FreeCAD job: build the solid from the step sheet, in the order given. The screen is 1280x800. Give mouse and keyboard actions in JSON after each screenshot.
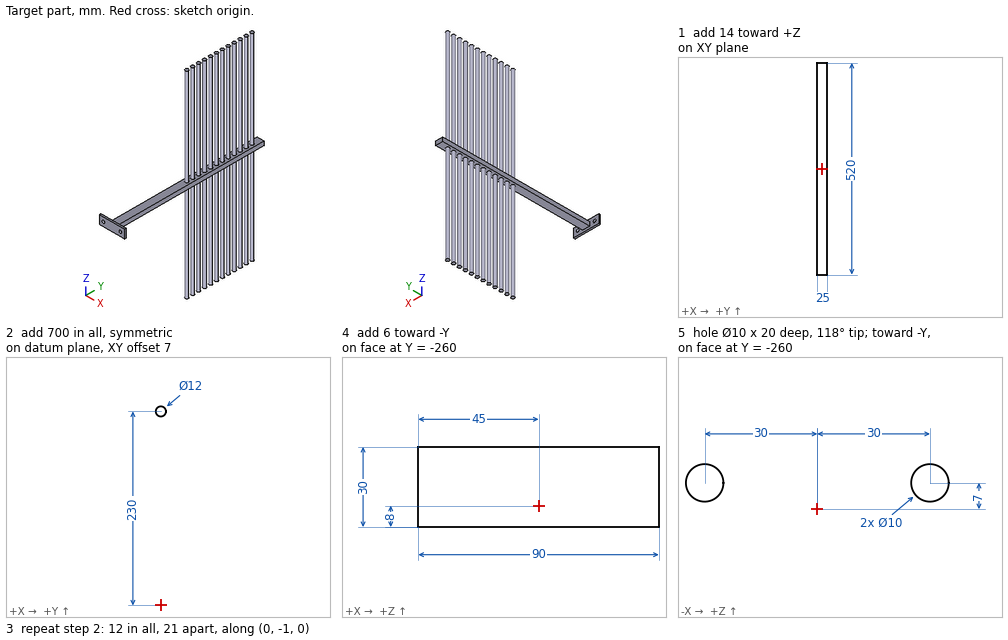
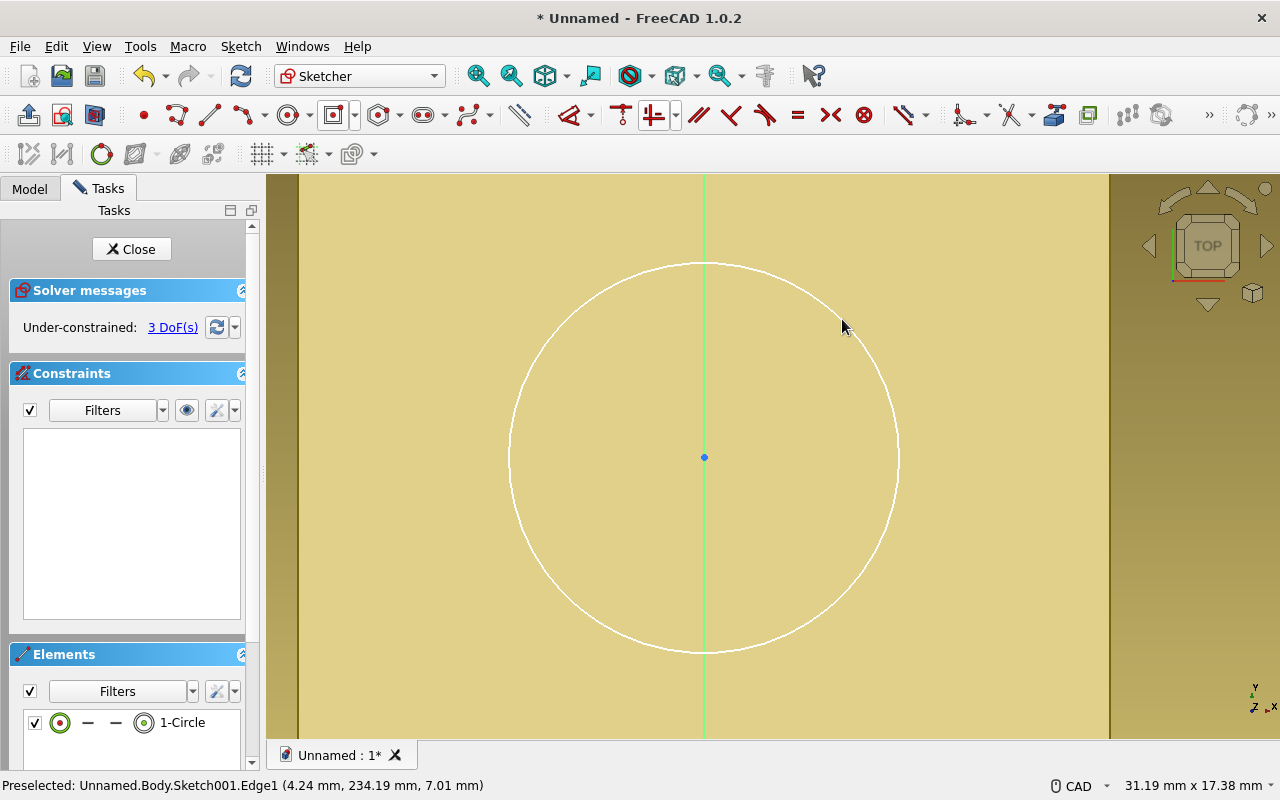
{"action": "left_click", "coordinate": [704, 458]}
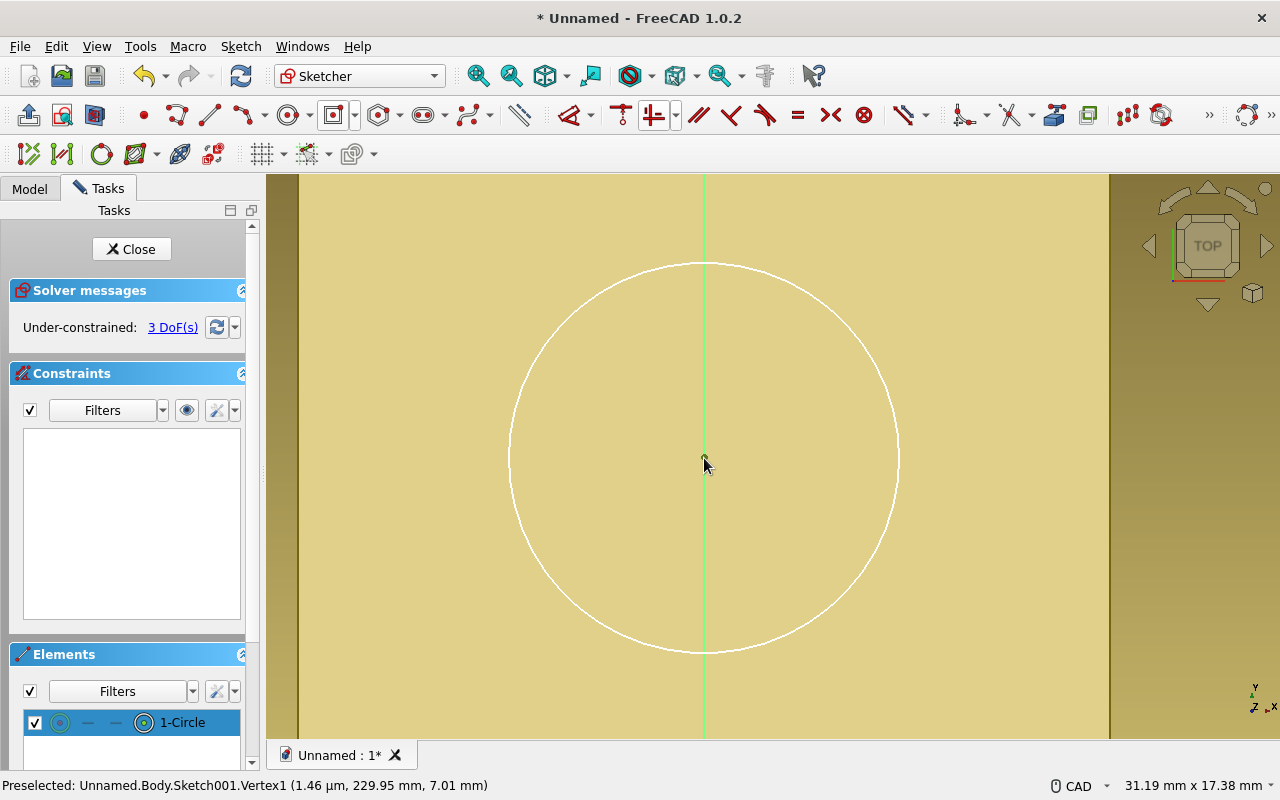
{"action": "left_click", "coordinate": [704, 602]}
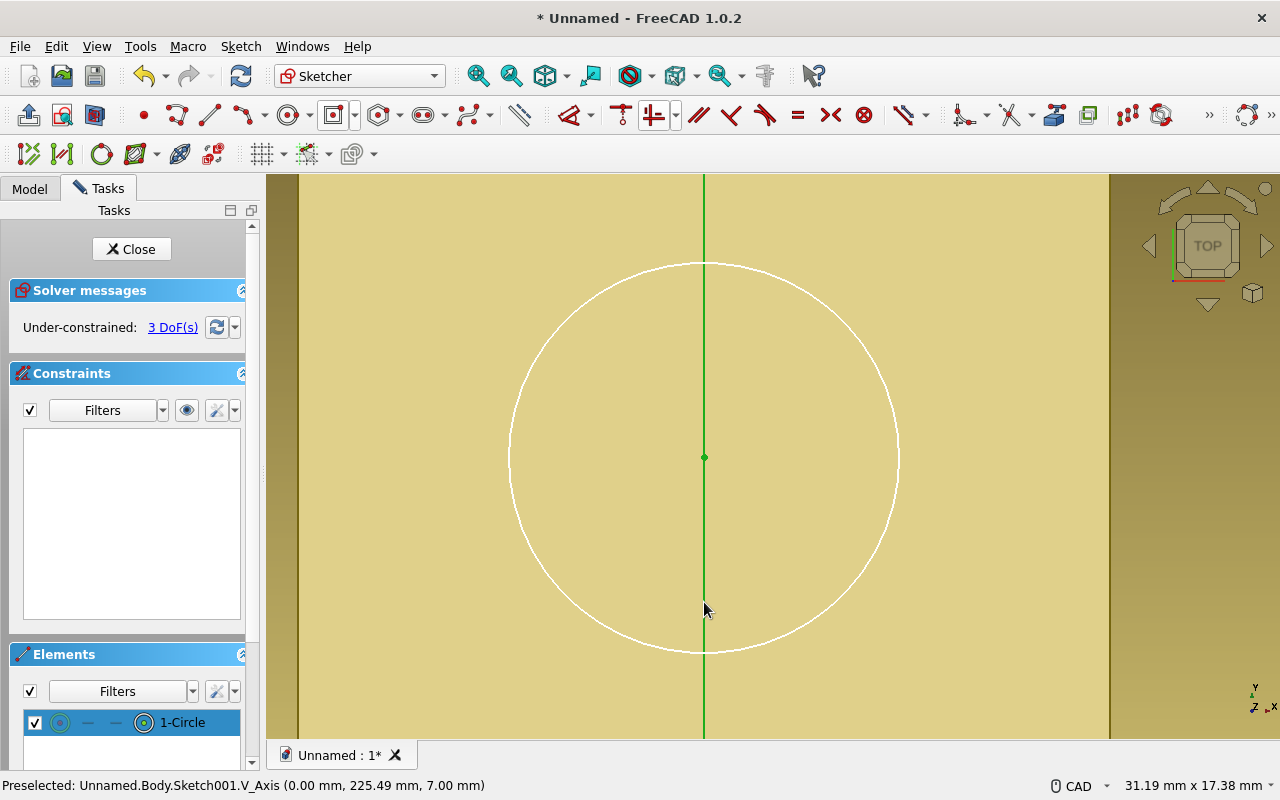
{"action": "left_click", "coordinate": [621, 116]}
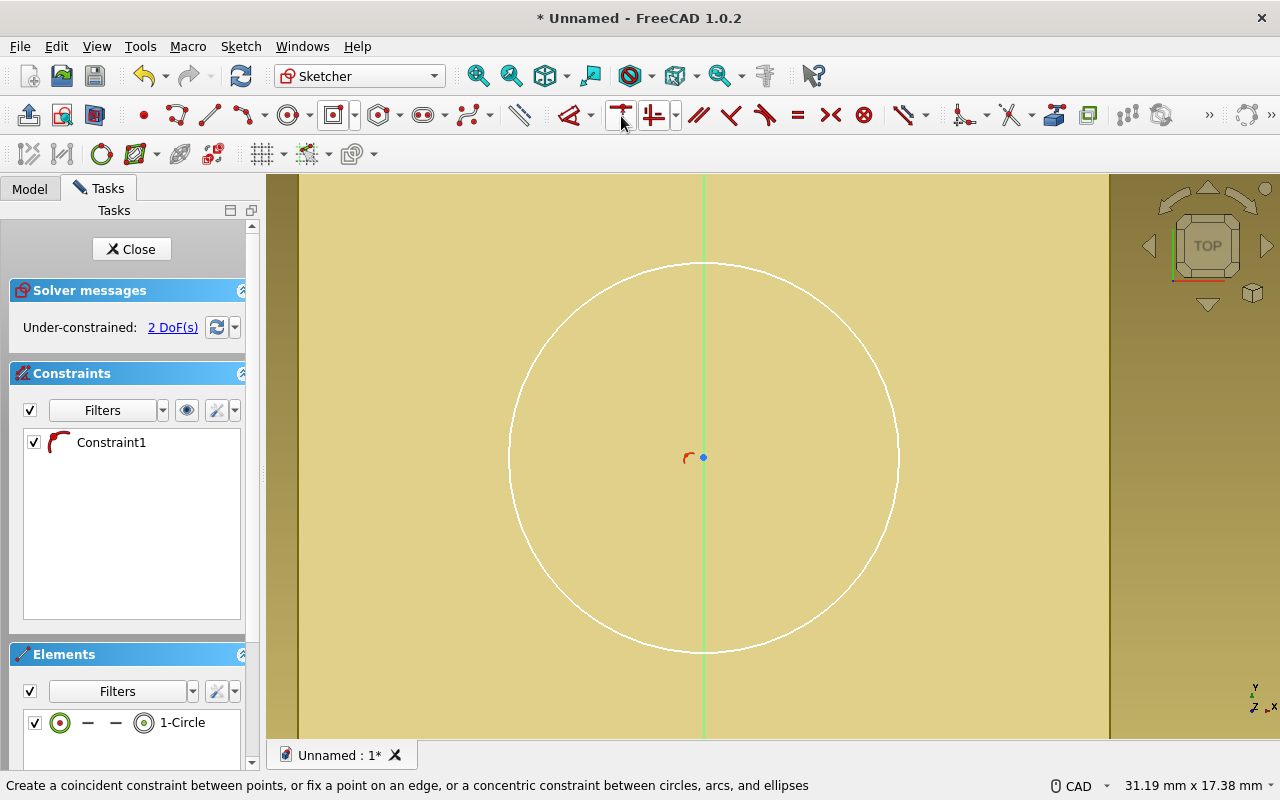
{"action": "left_click", "coordinate": [568, 116]}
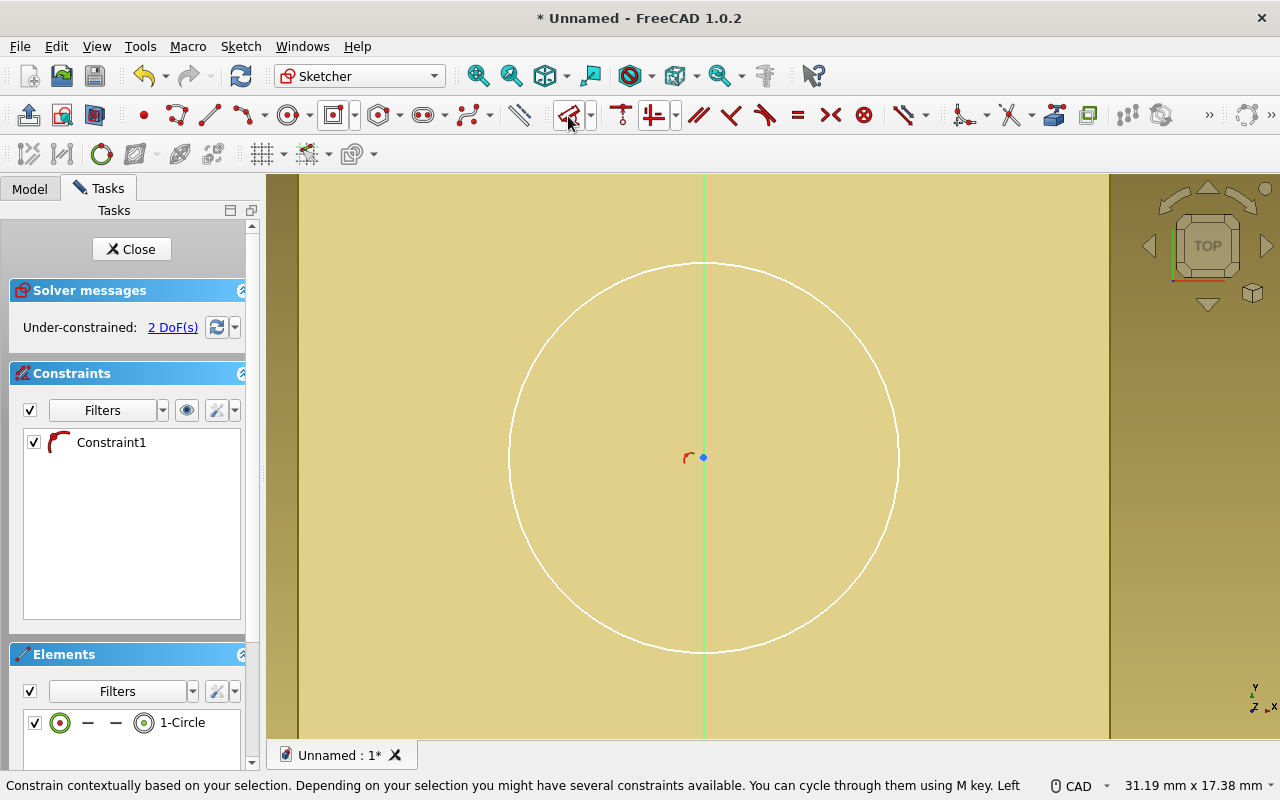
{"action": "left_click", "coordinate": [842, 320]}
{"action": "left_click", "coordinate": [865, 297]}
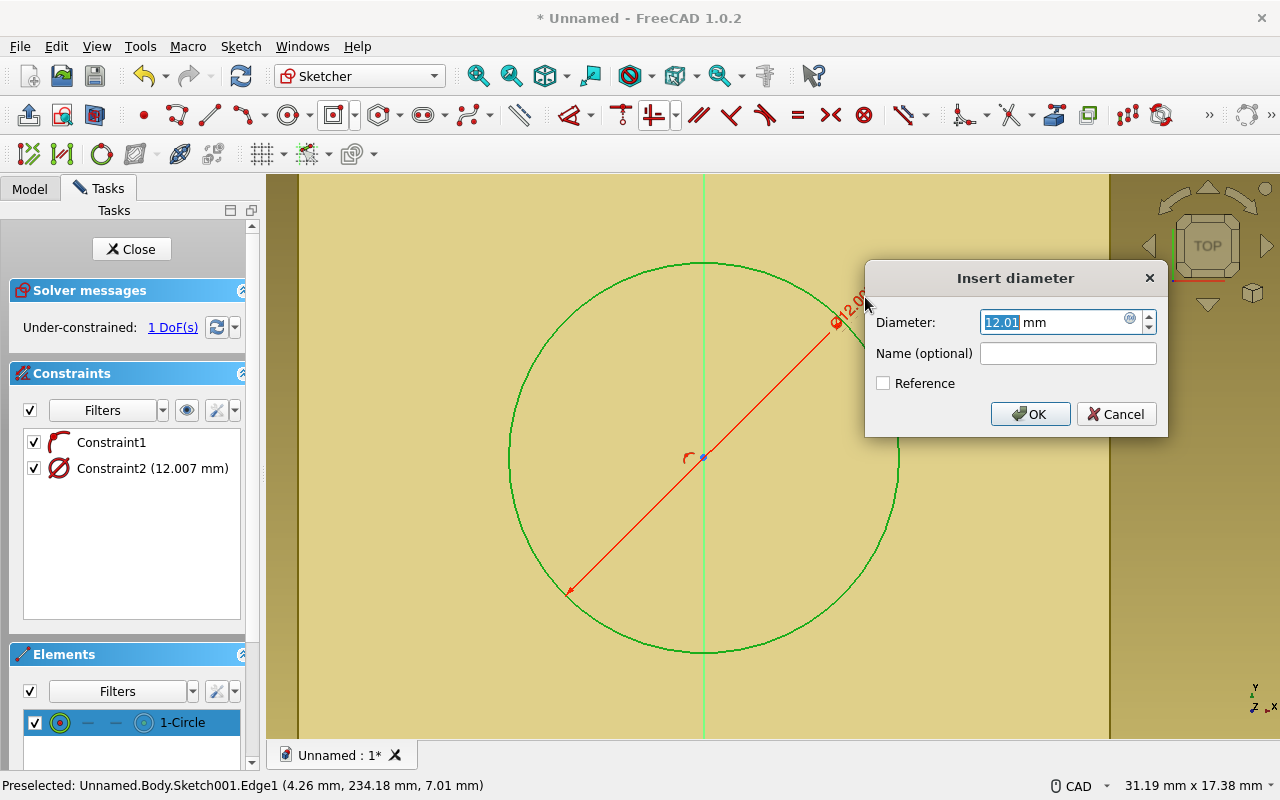
{"action": "type", "text": "12"}
{"action": "key", "text": "Return"}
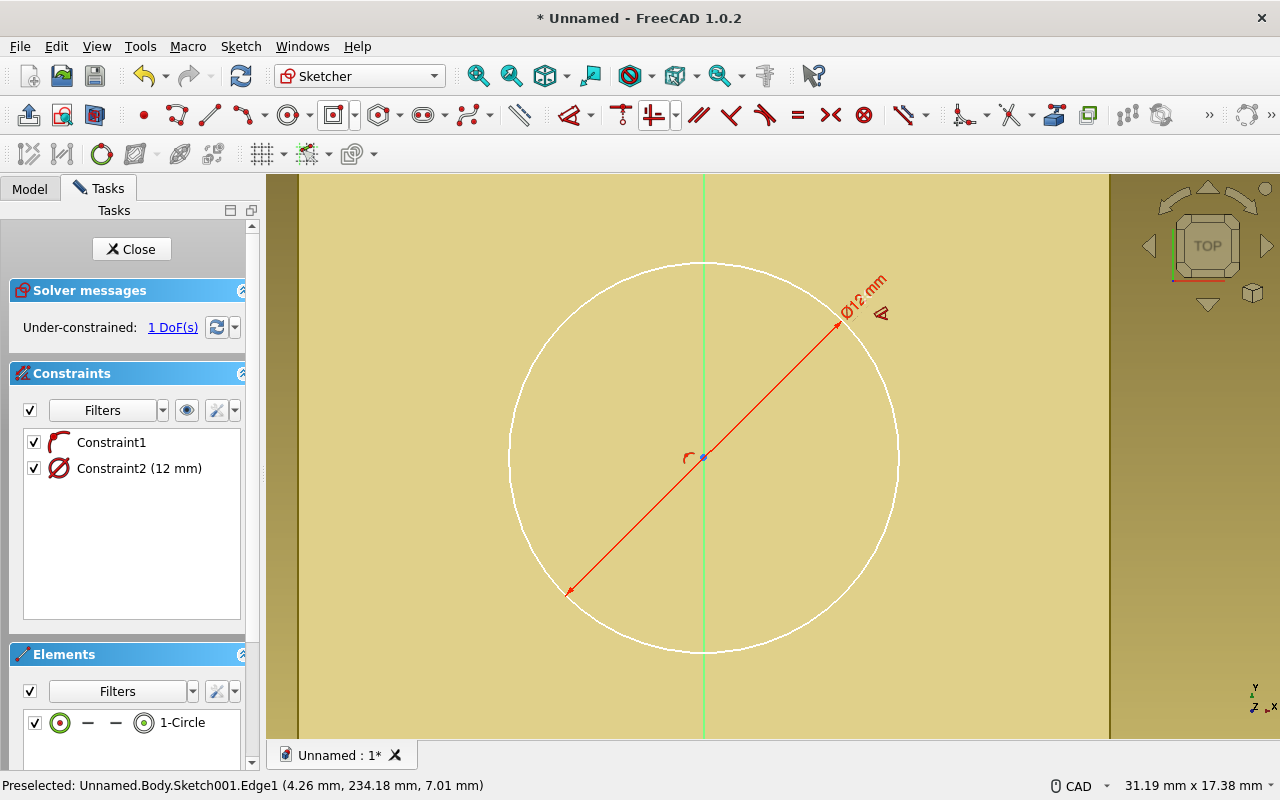
{"action": "left_click", "coordinate": [704, 458]}
{"action": "left_click", "coordinate": [738, 585]}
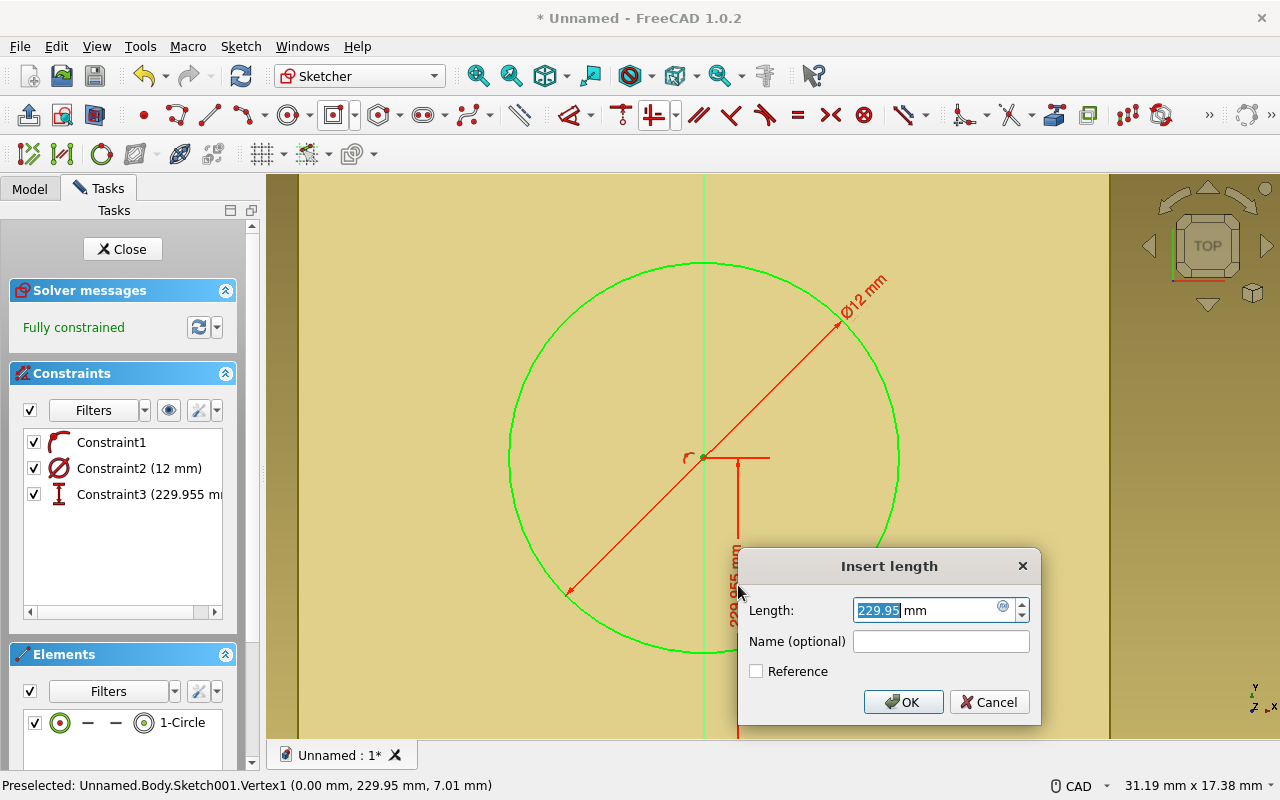
{"action": "type", "text": "230"}
{"action": "key", "text": "Return"}
{"action": "key", "text": "Escape"}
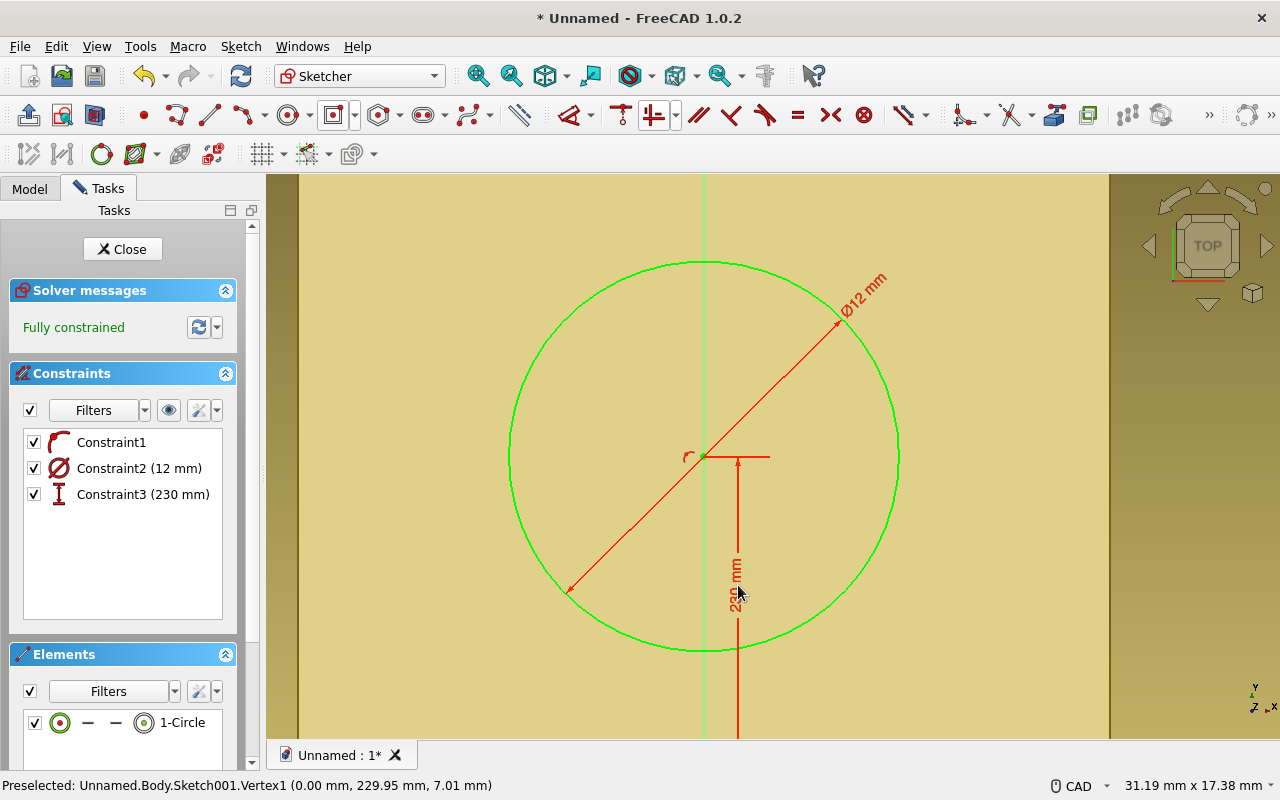
{"action": "left_click", "coordinate": [123, 249]}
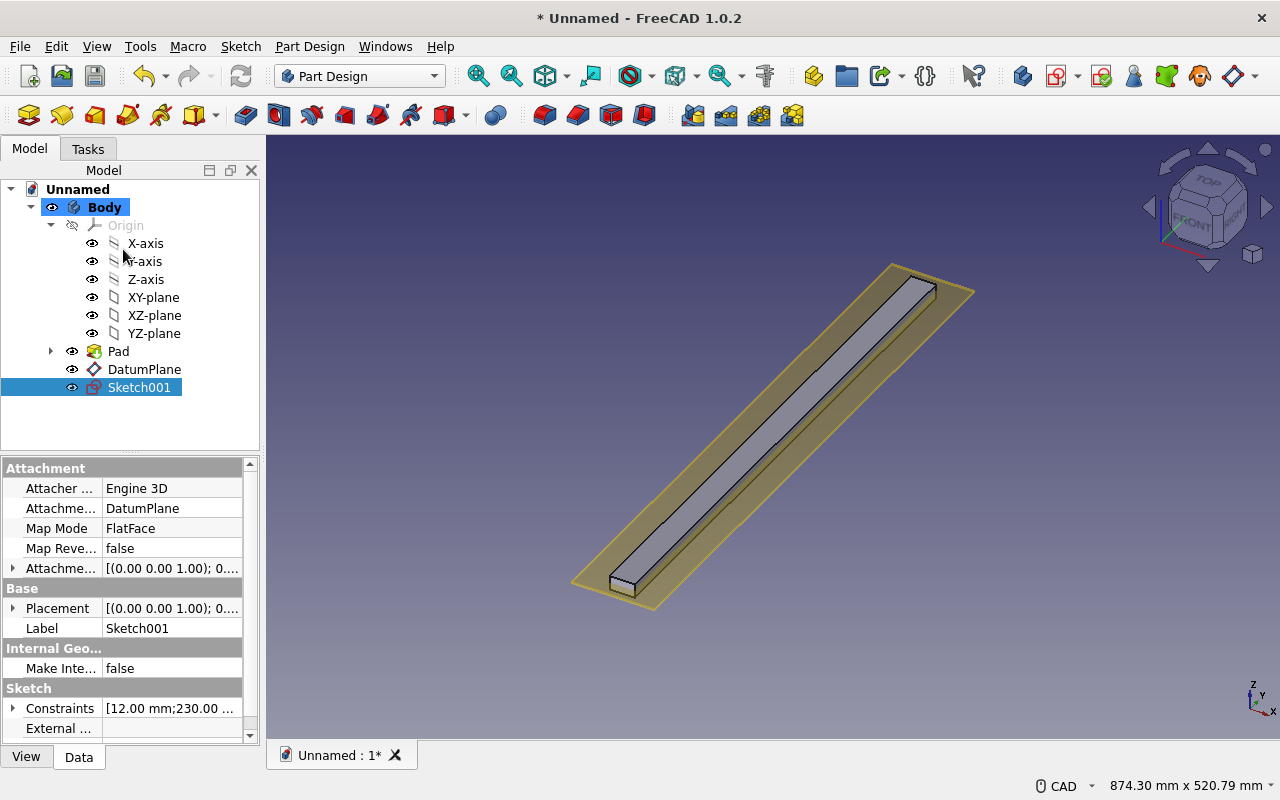
{"action": "left_click", "coordinate": [29, 116]}